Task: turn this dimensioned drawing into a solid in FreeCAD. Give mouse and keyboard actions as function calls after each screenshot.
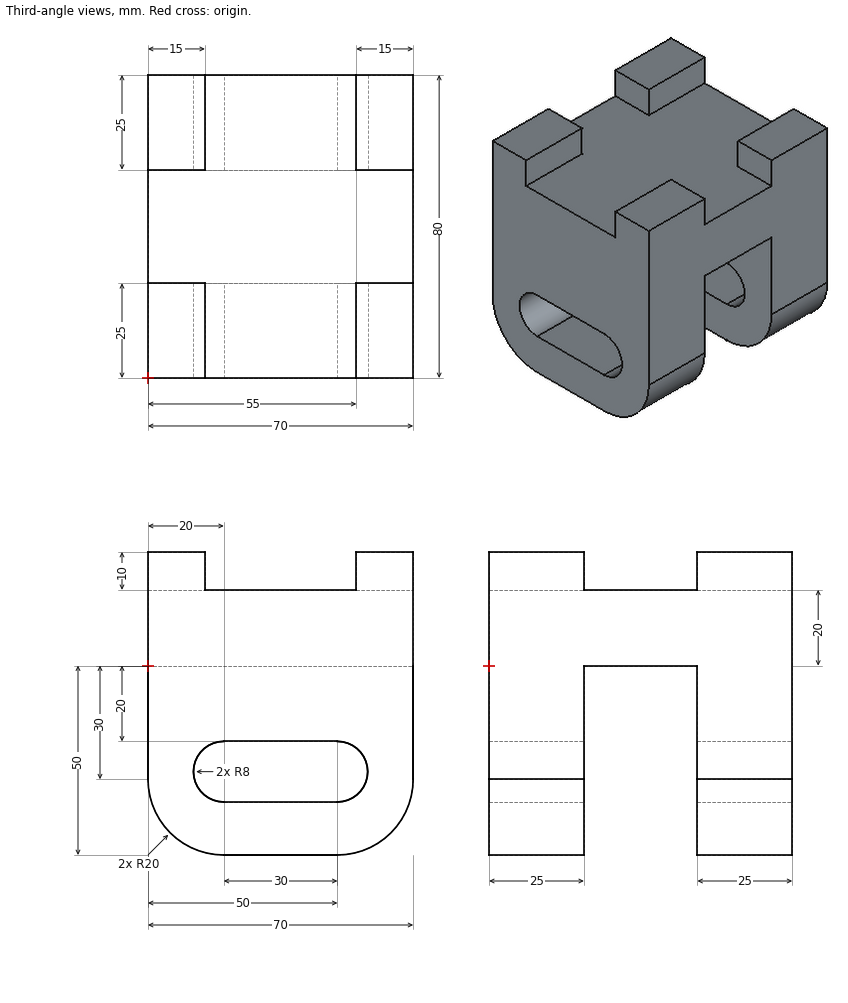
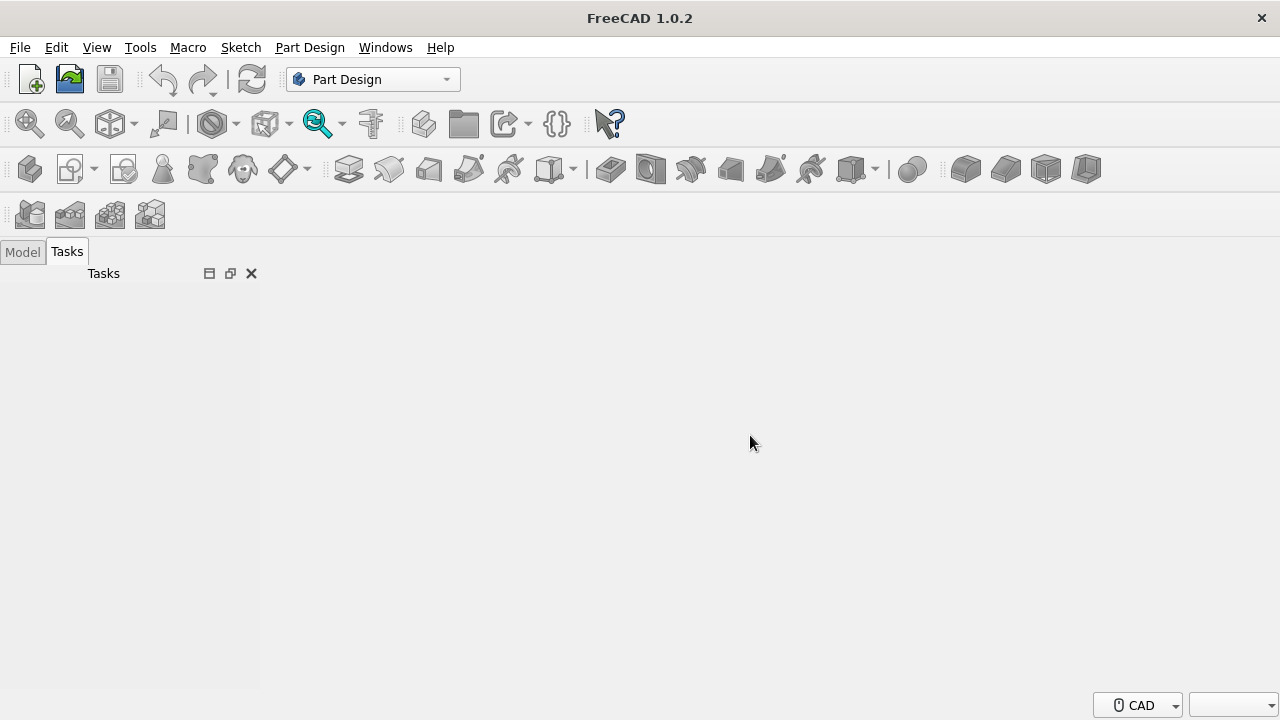
click(30, 80)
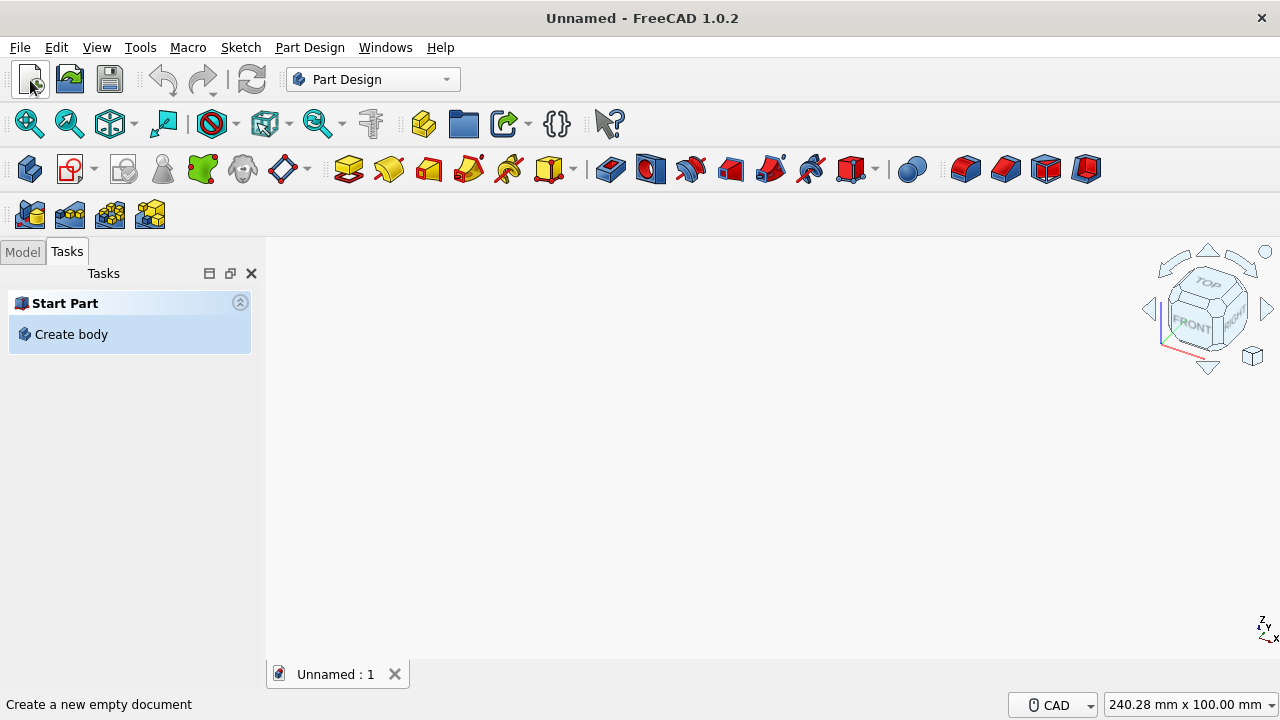
click(70, 170)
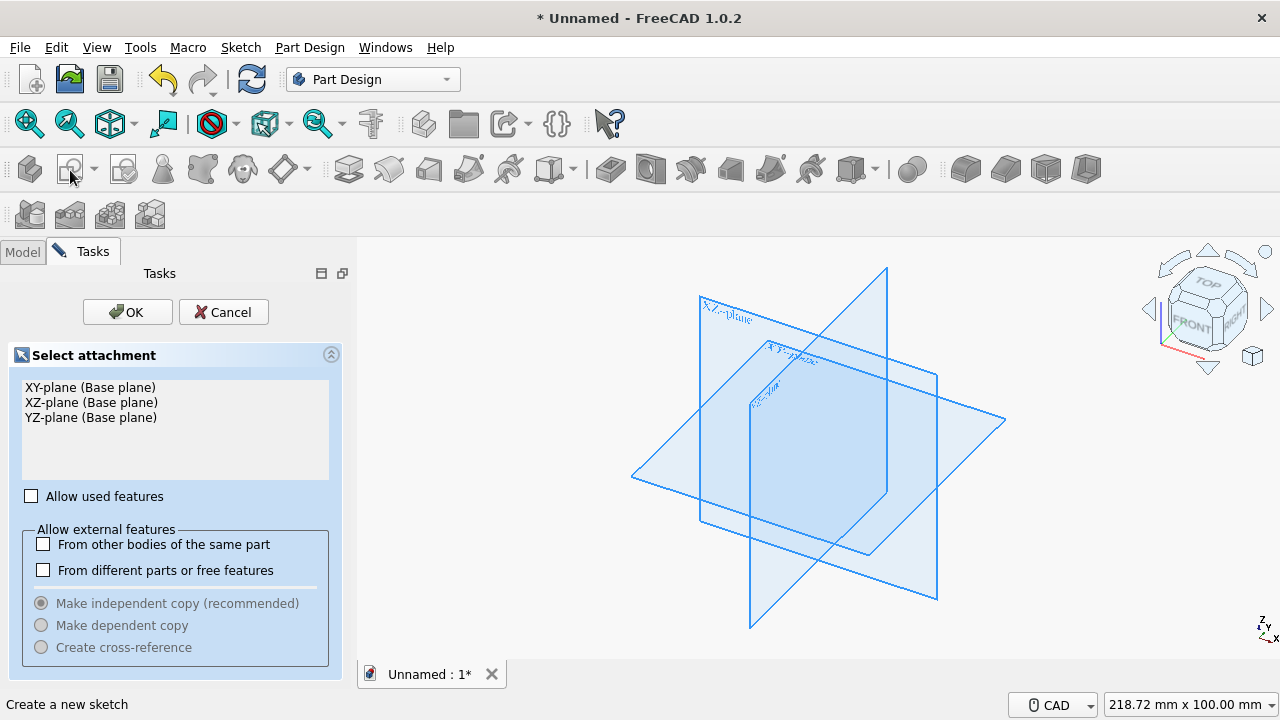
click(82, 388)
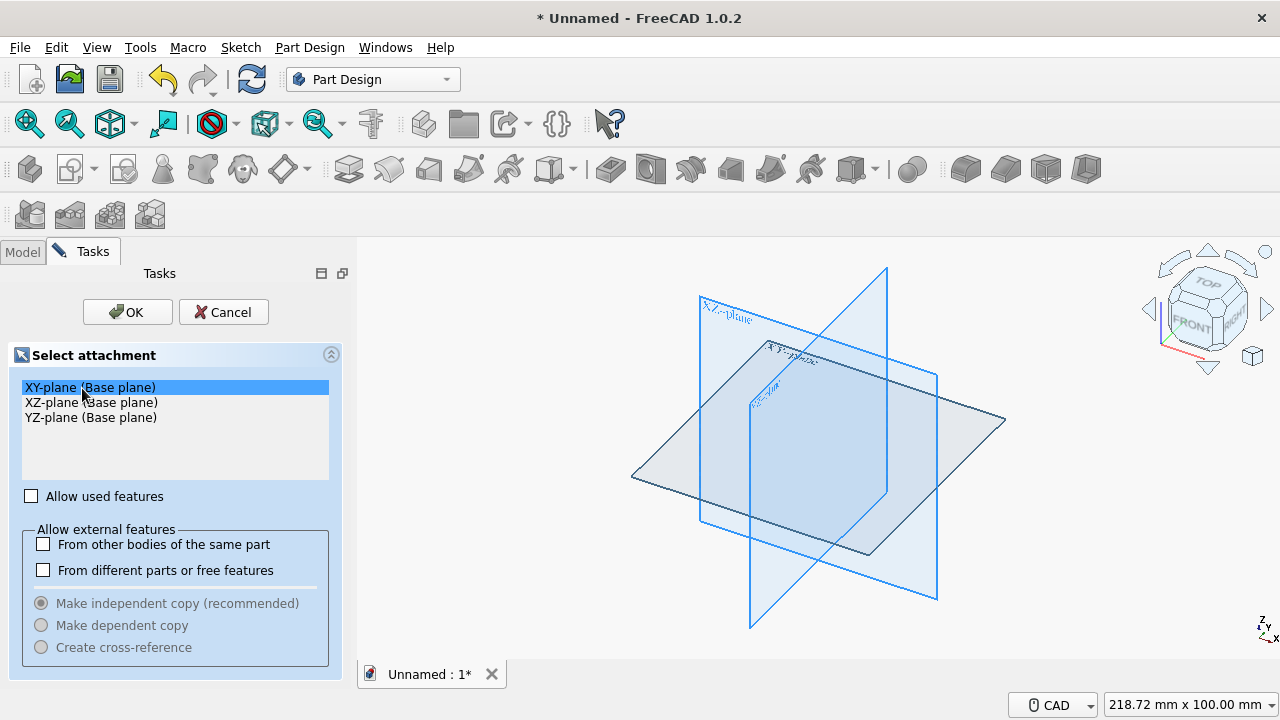
click(128, 312)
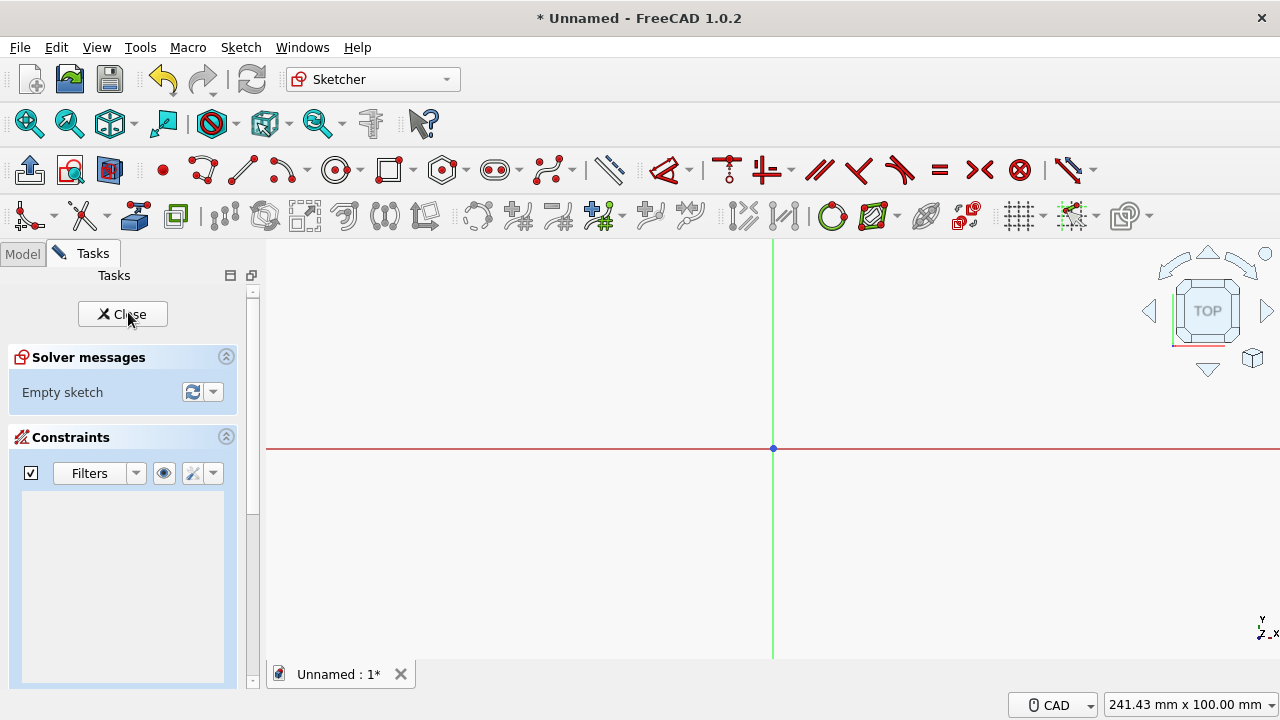
scroll(442, 631, down, 3)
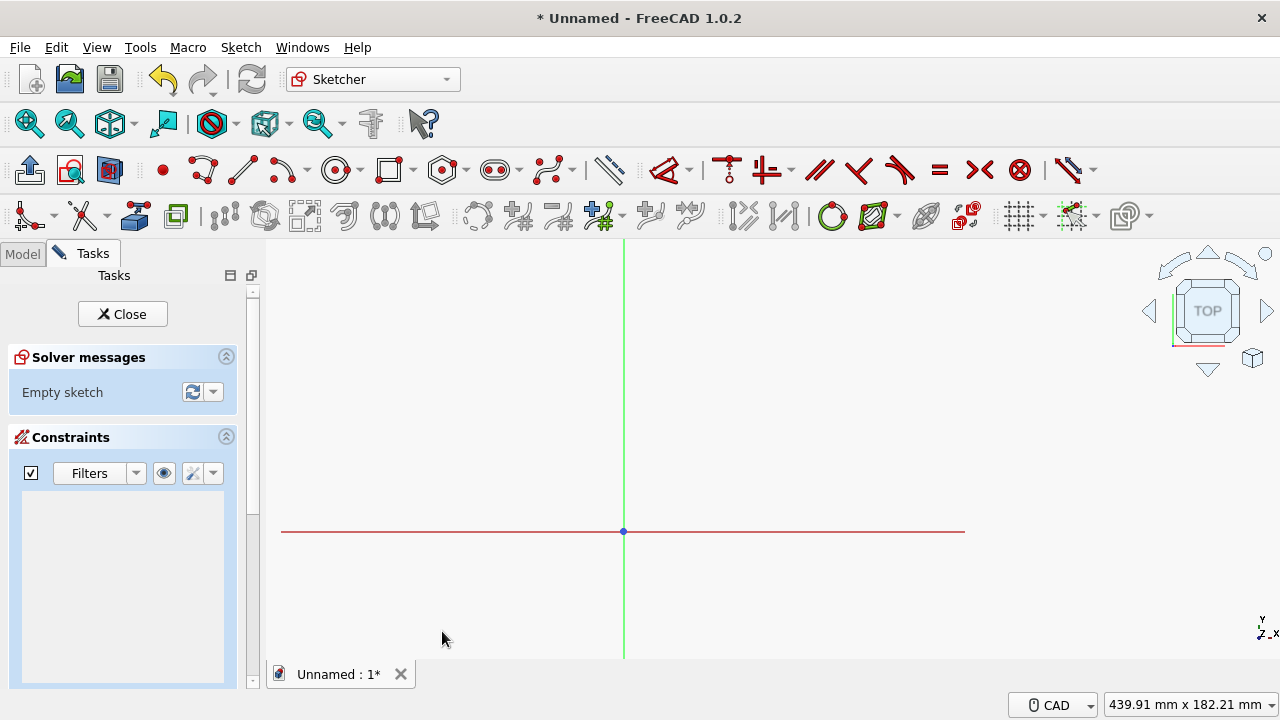
scroll(704, 420, up, 2)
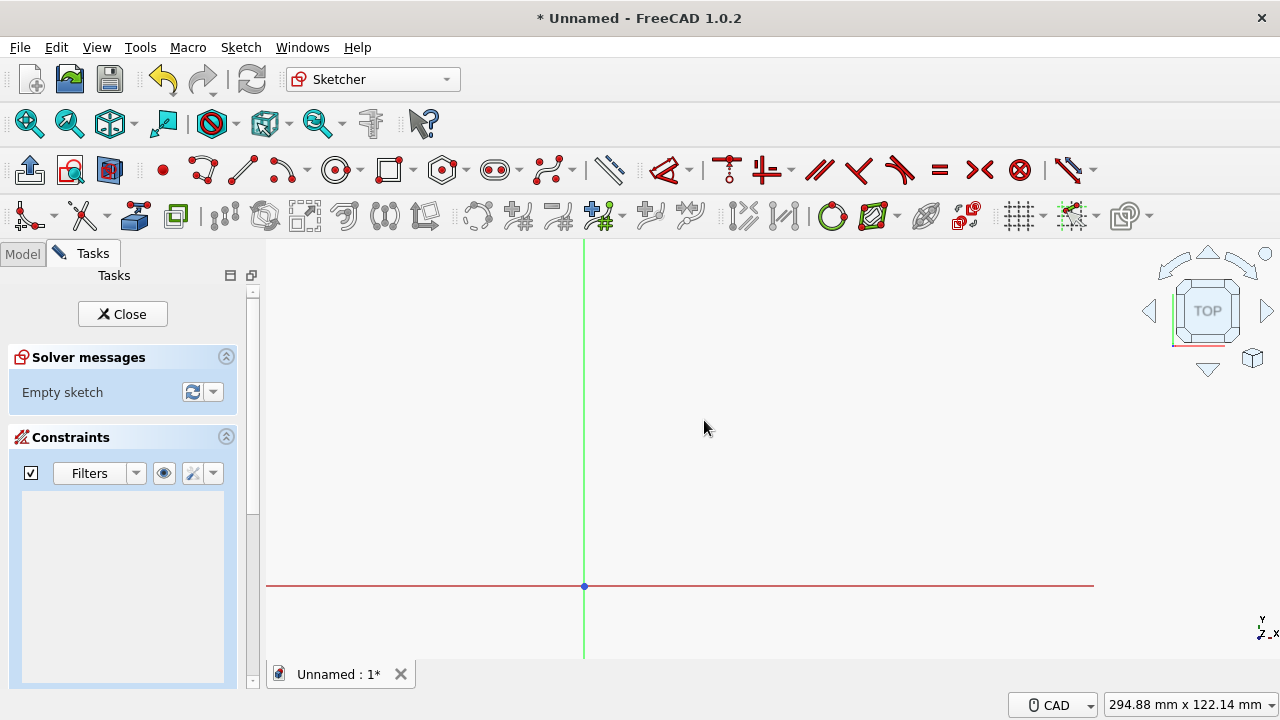
click(390, 170)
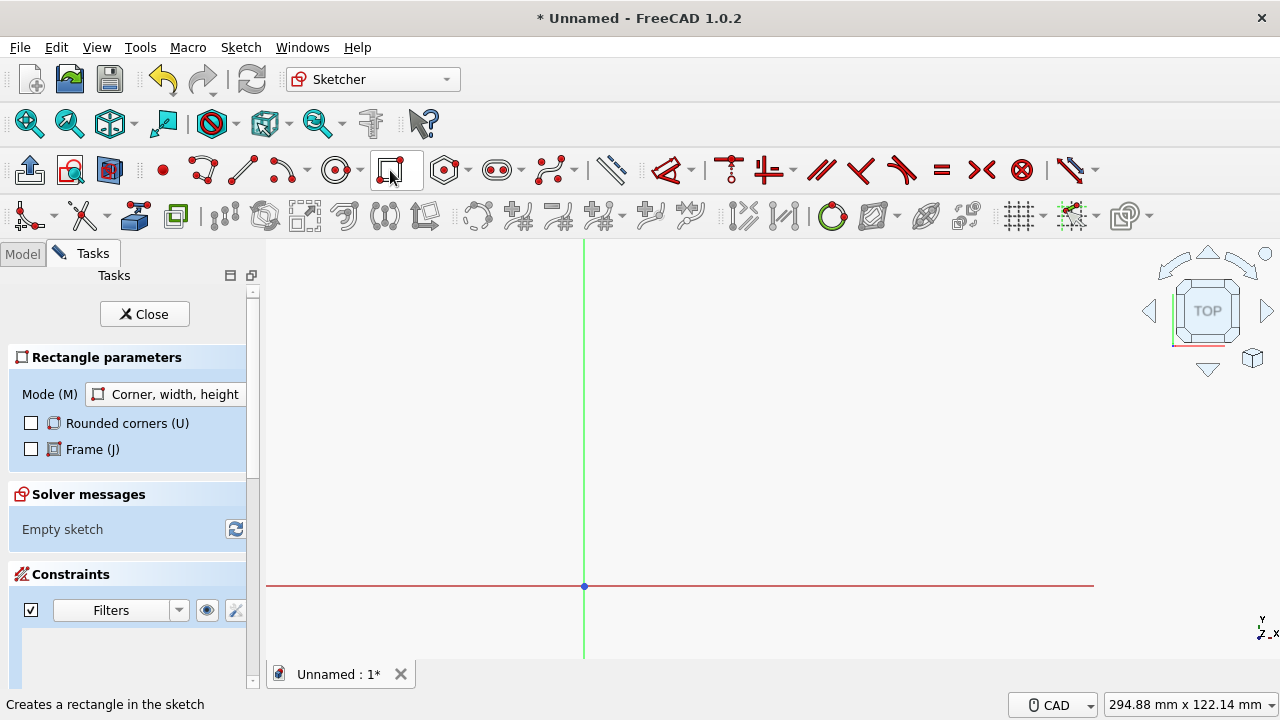
click(584, 586)
move(825, 311)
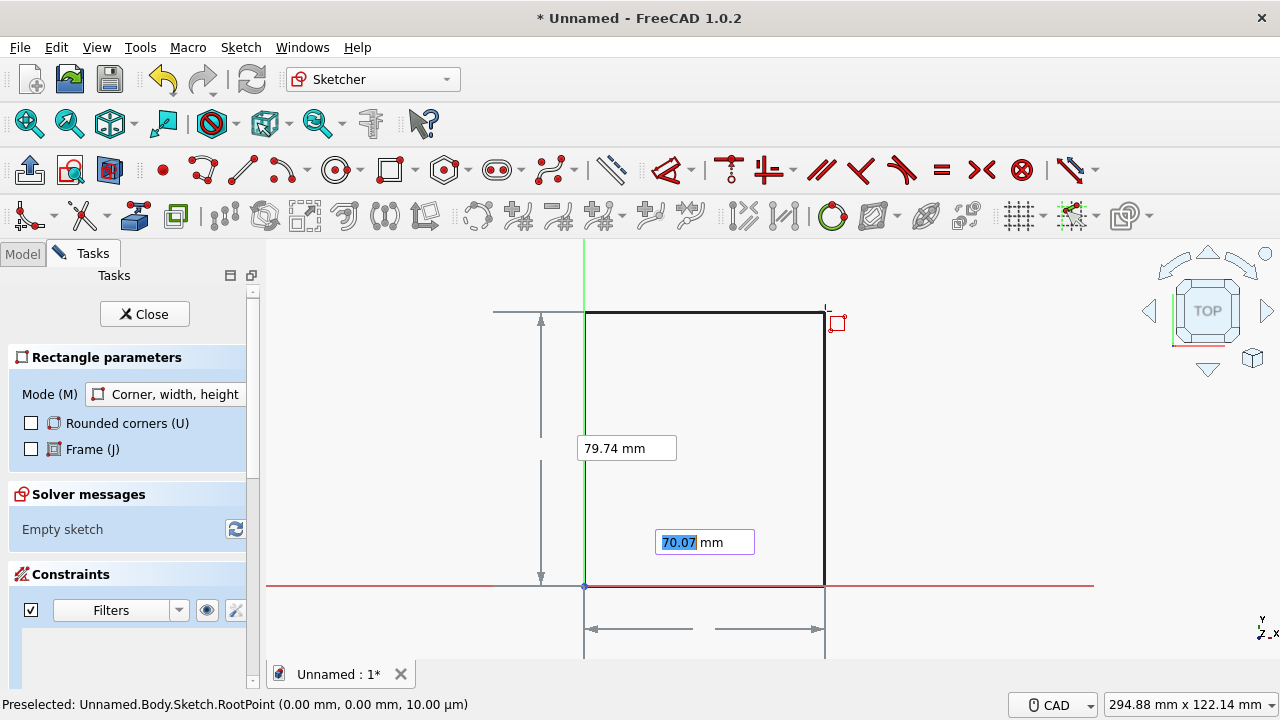
text(70)
key(Tab)
text(80)
key(Return)
key(Escape)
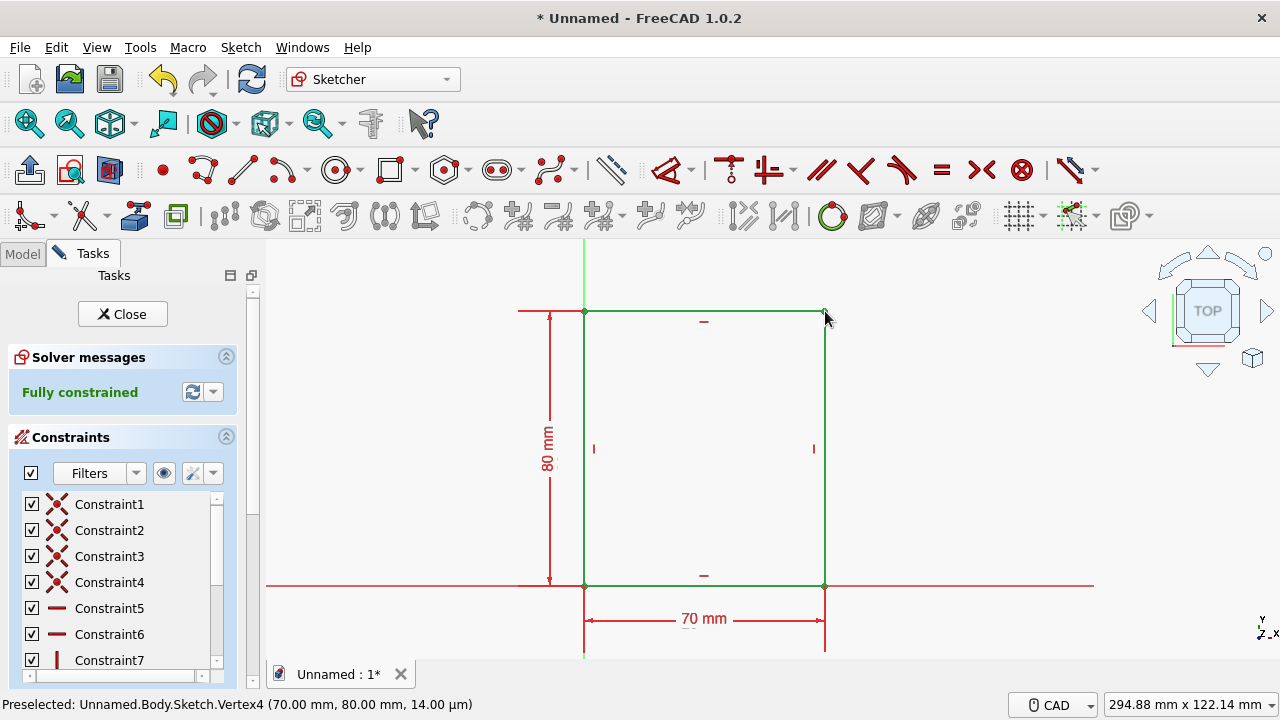
click(123, 314)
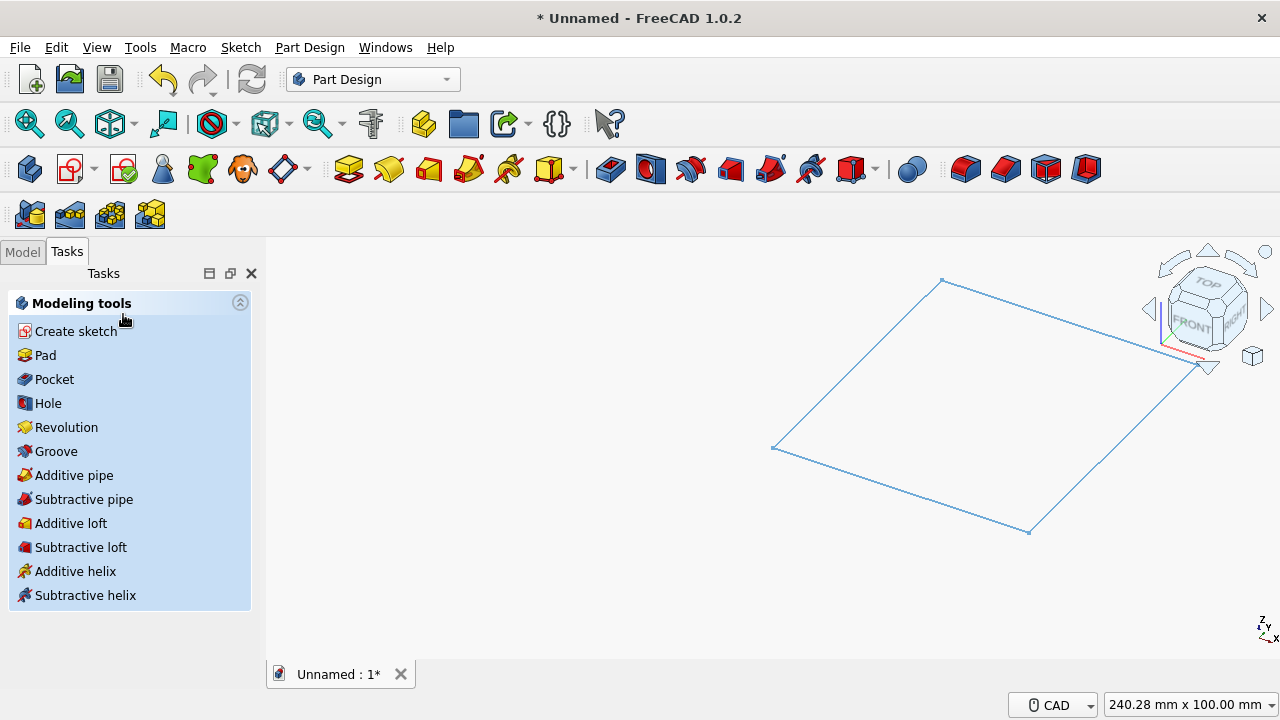
click(350, 170)